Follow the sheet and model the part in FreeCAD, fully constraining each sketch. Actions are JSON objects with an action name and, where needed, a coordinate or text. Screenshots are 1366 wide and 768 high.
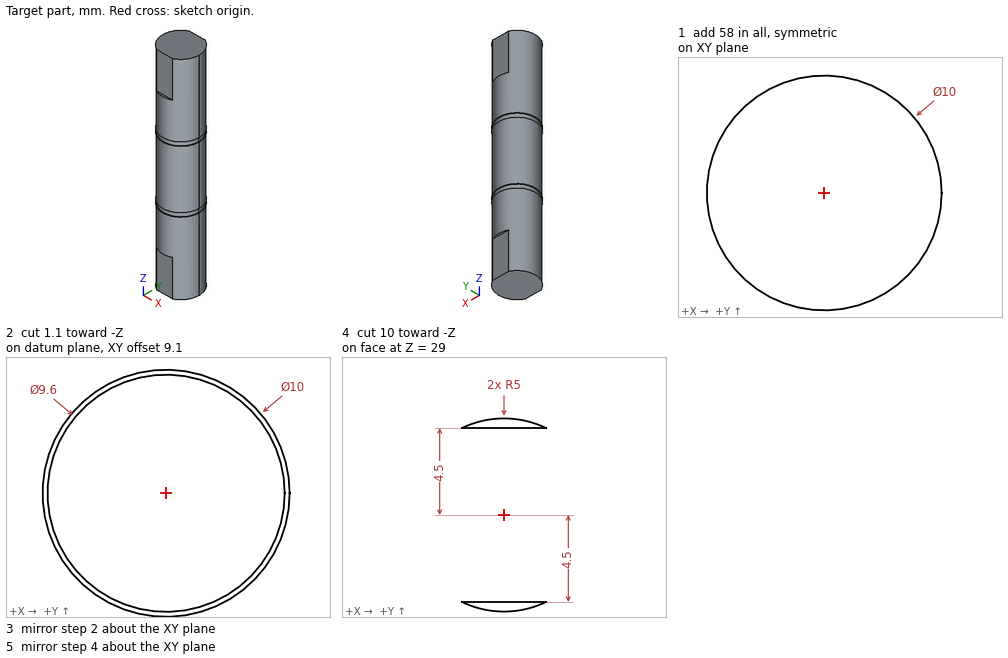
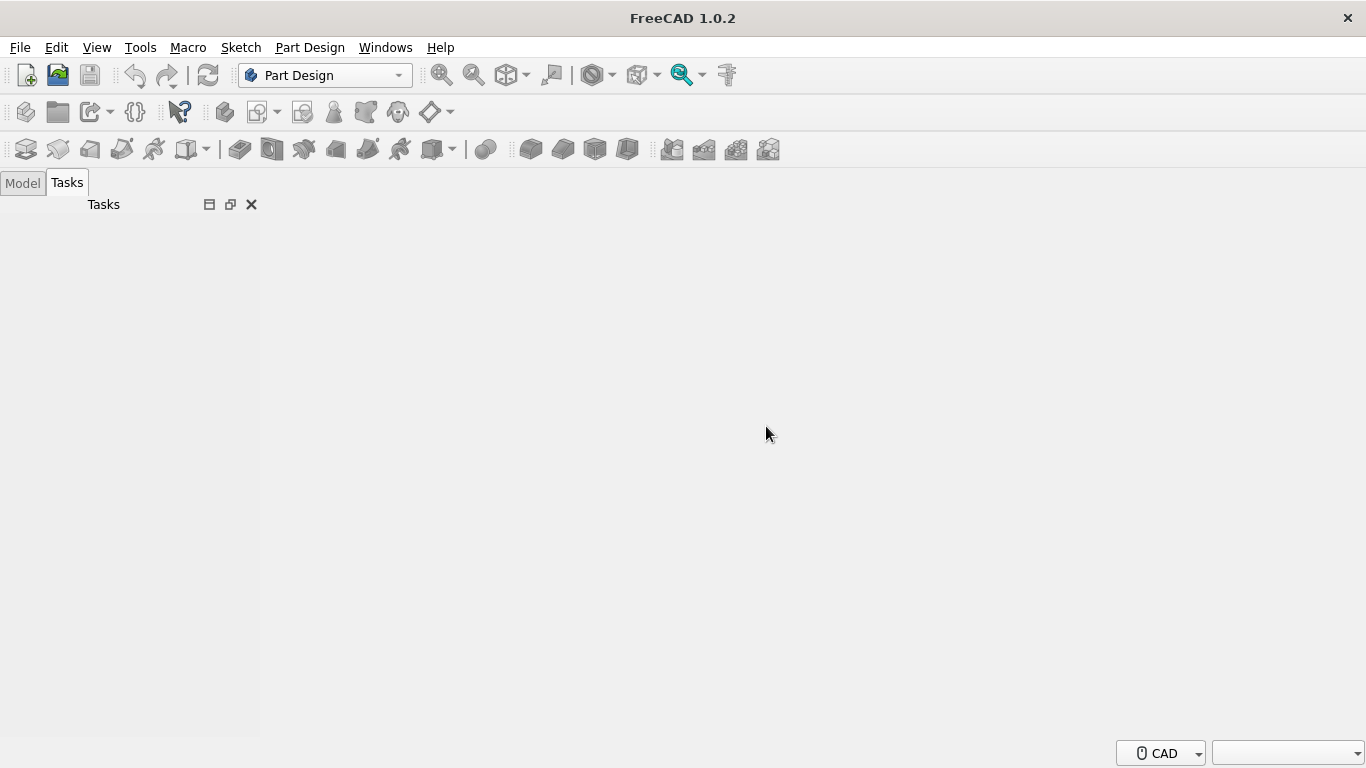
{"action": "key", "text": "ctrl+n"}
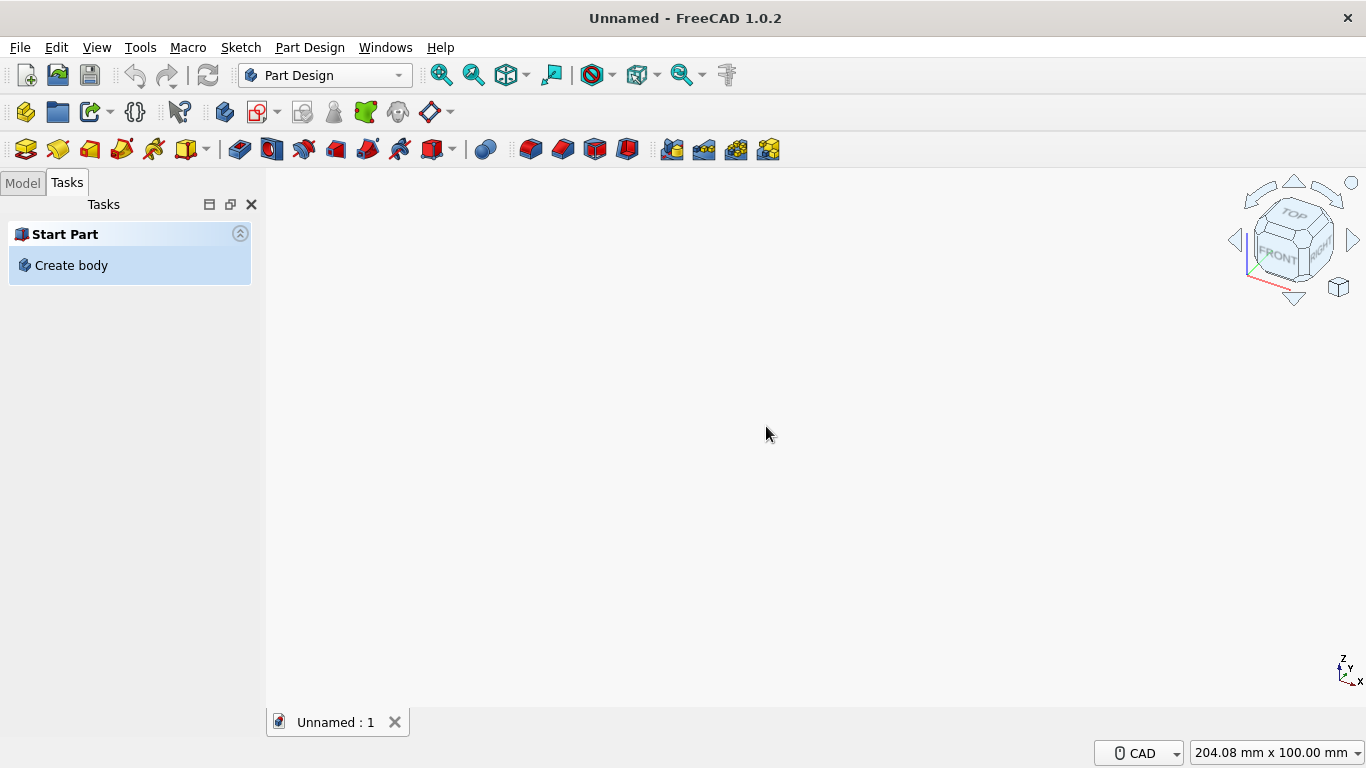
{"action": "left_click", "coordinate": [258, 112]}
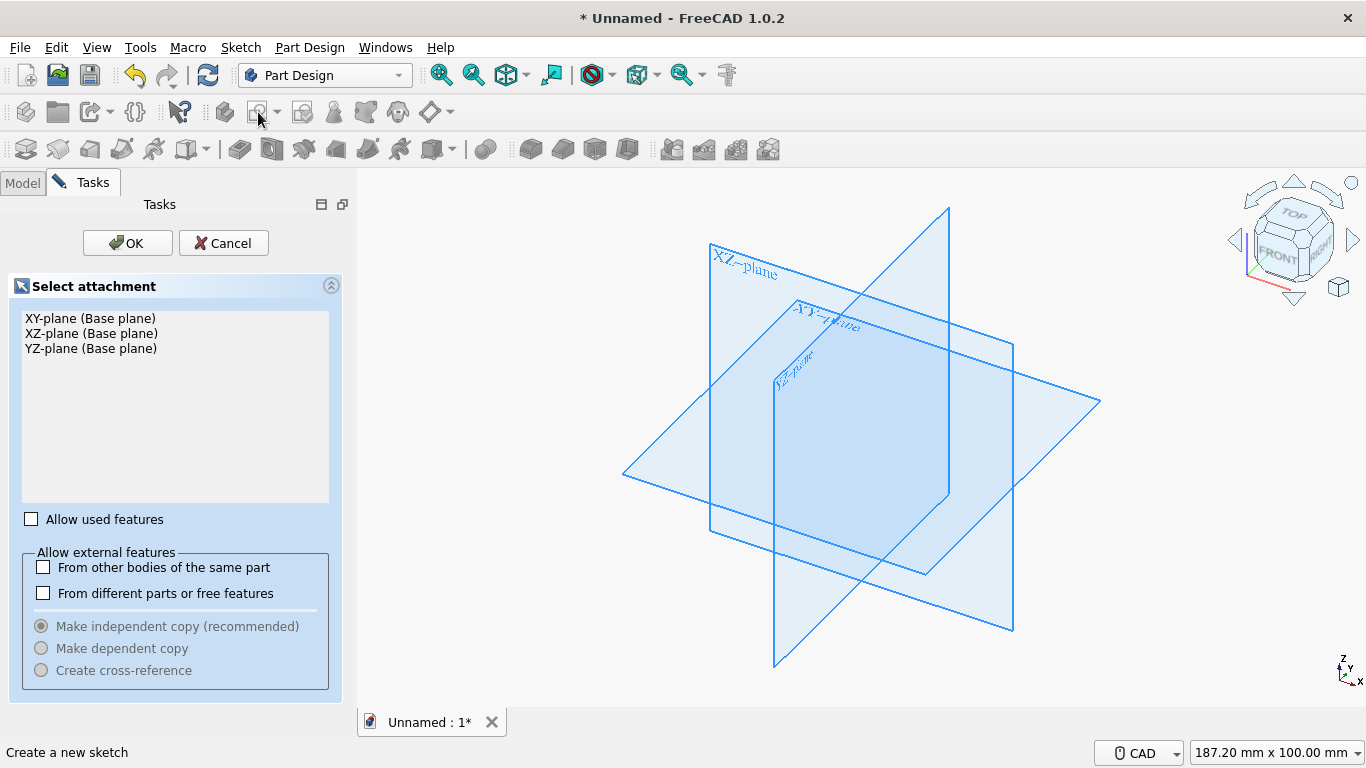
{"action": "left_click", "coordinate": [82, 318]}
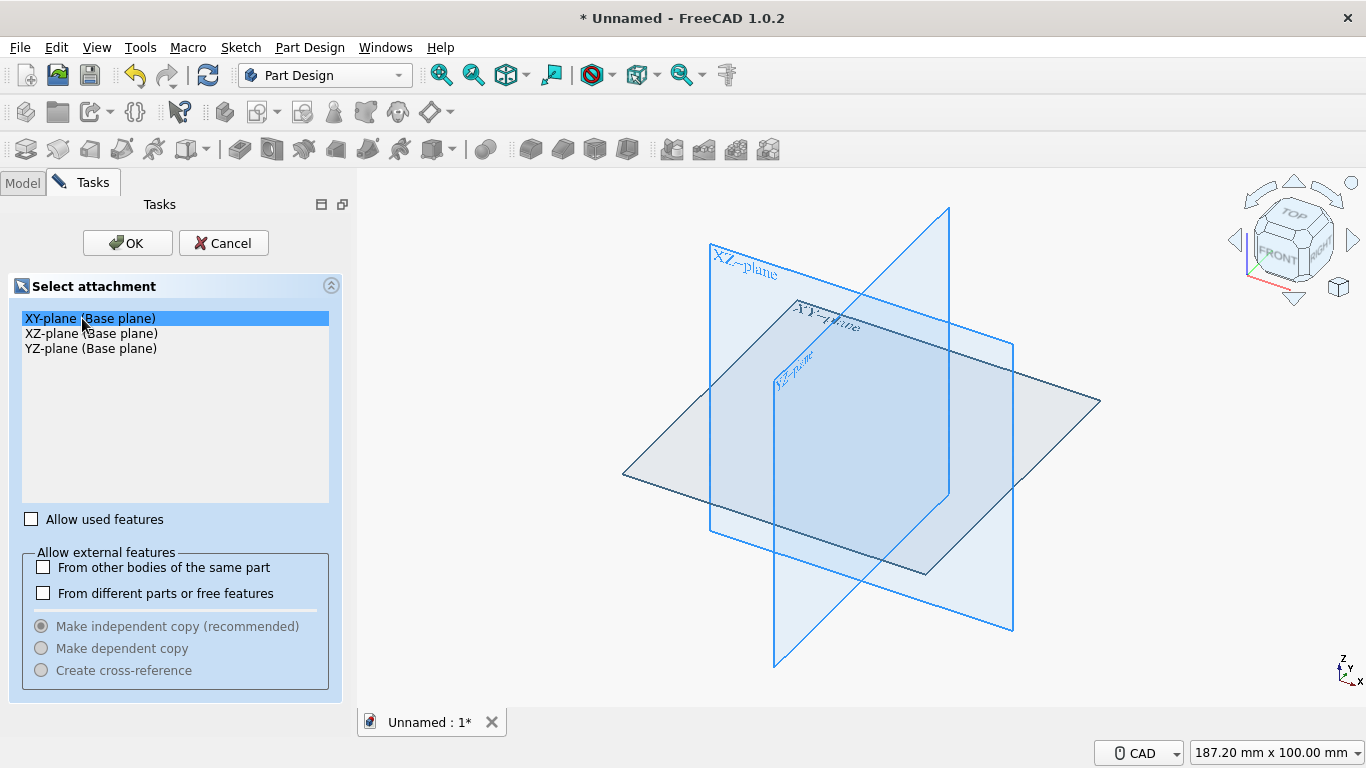
{"action": "left_click", "coordinate": [128, 243]}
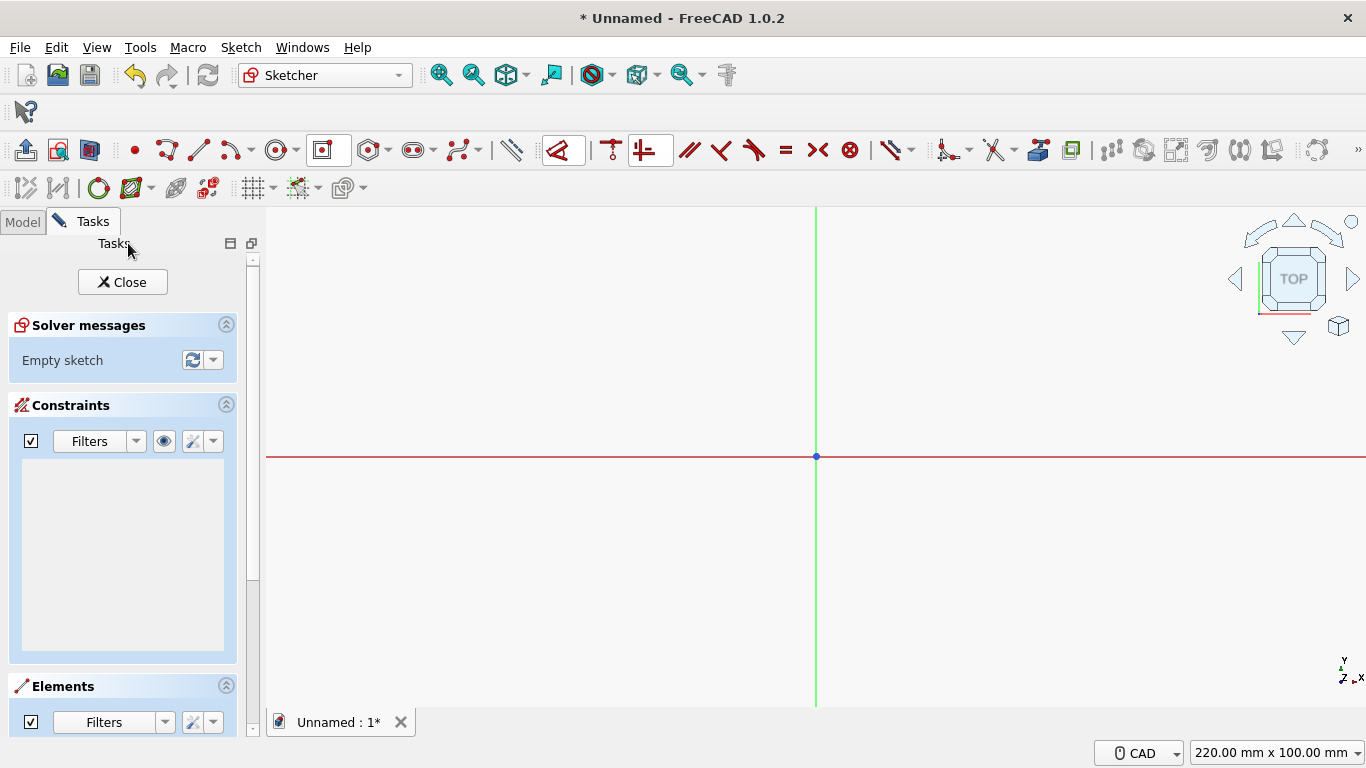
{"action": "scroll", "coordinate": [830, 457], "scroll_direction": "up", "scroll_amount": 9}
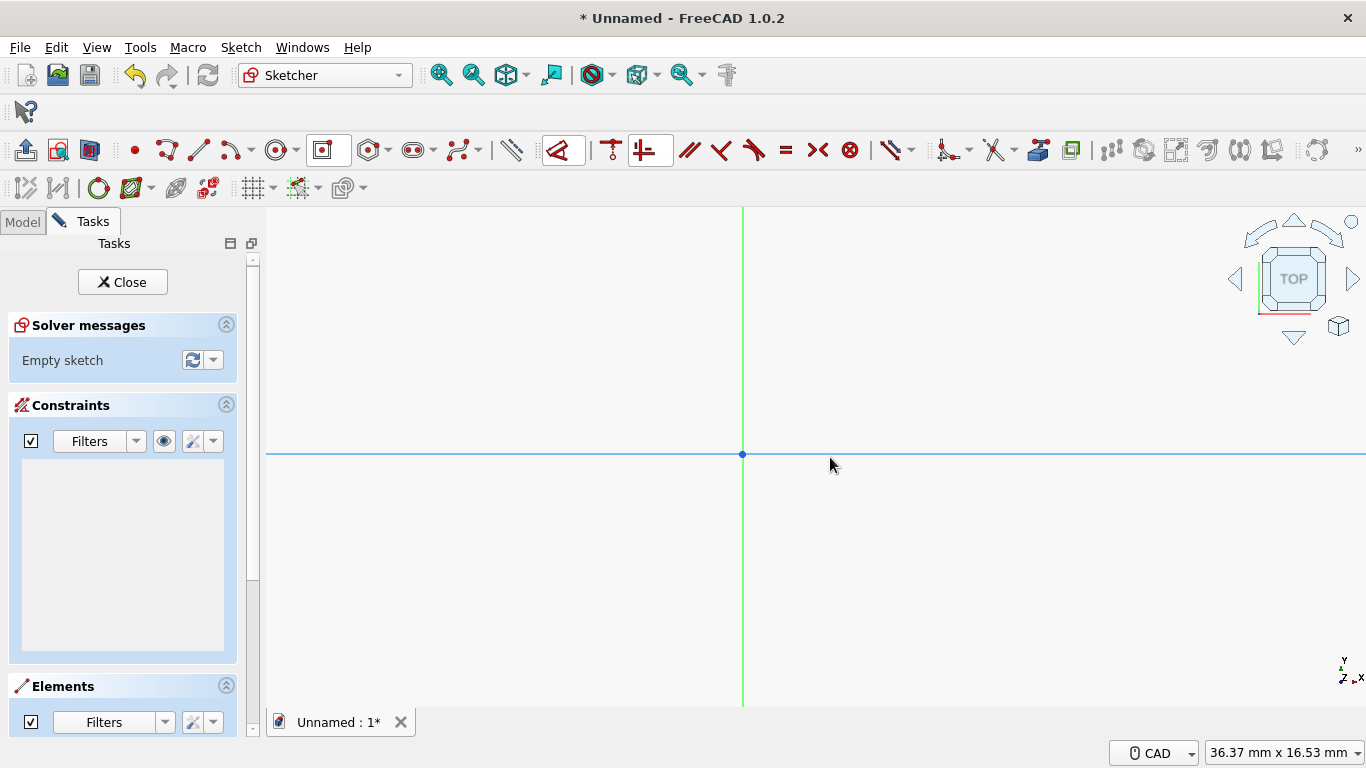
{"action": "left_click", "coordinate": [276, 150]}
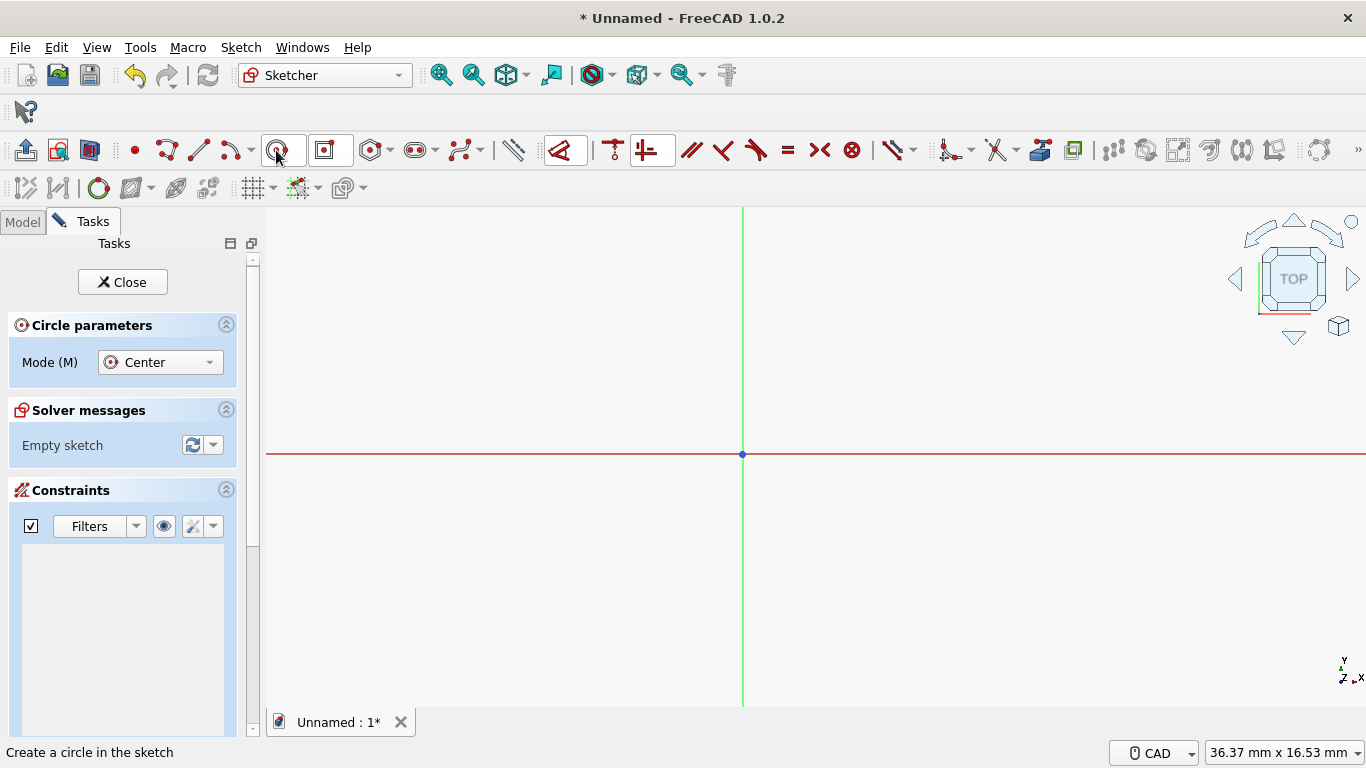
{"action": "left_click", "coordinate": [743, 454]}
{"action": "left_click", "coordinate": [850, 348]}
{"action": "key", "text": "Escape"}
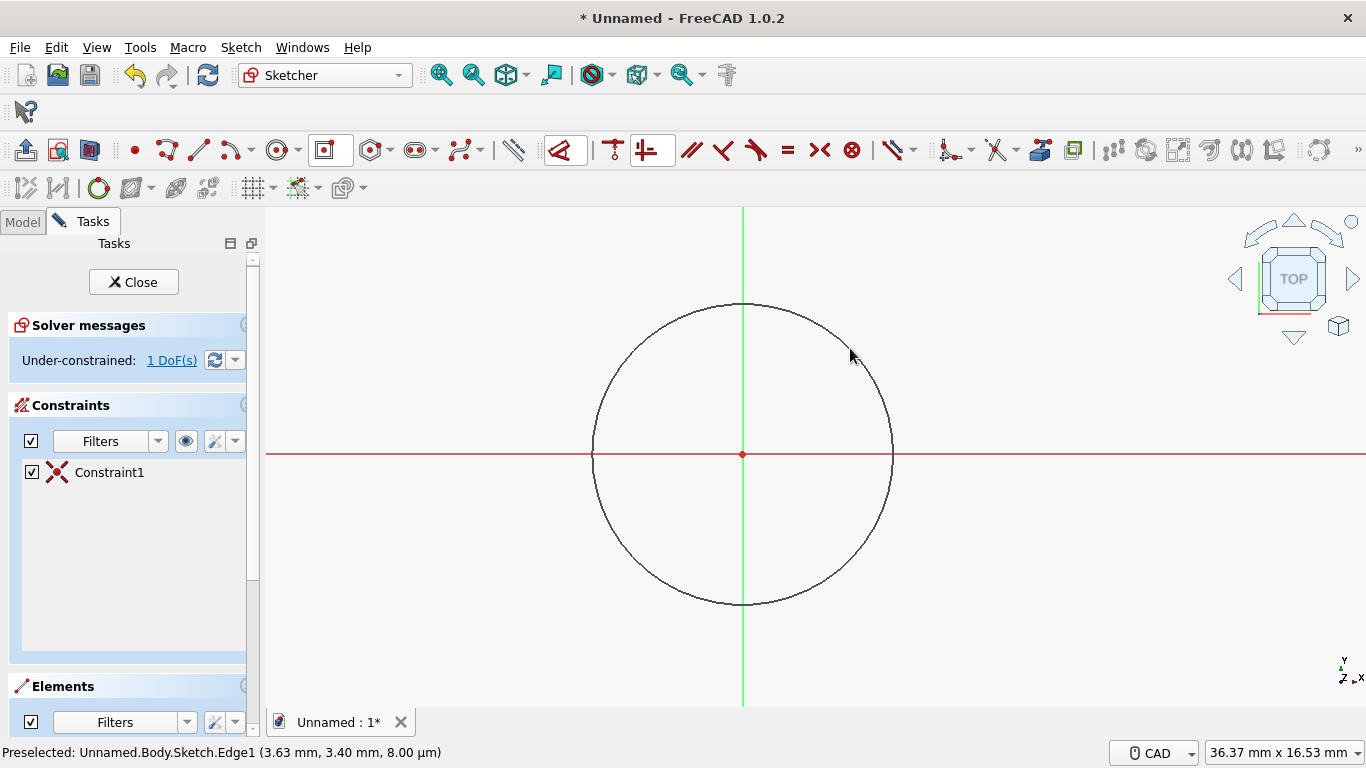
{"action": "left_click", "coordinate": [560, 150]}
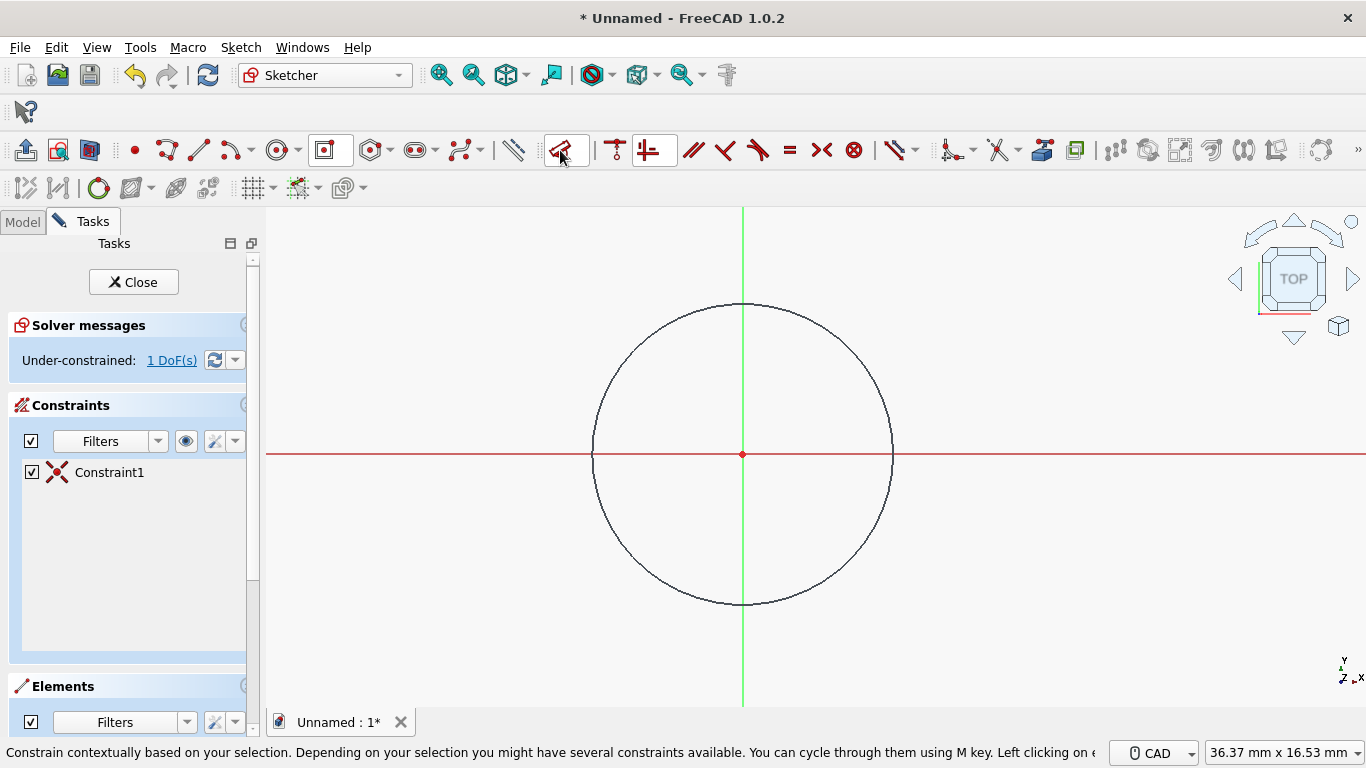
{"action": "left_click", "coordinate": [849, 348]}
{"action": "left_click", "coordinate": [872, 325]}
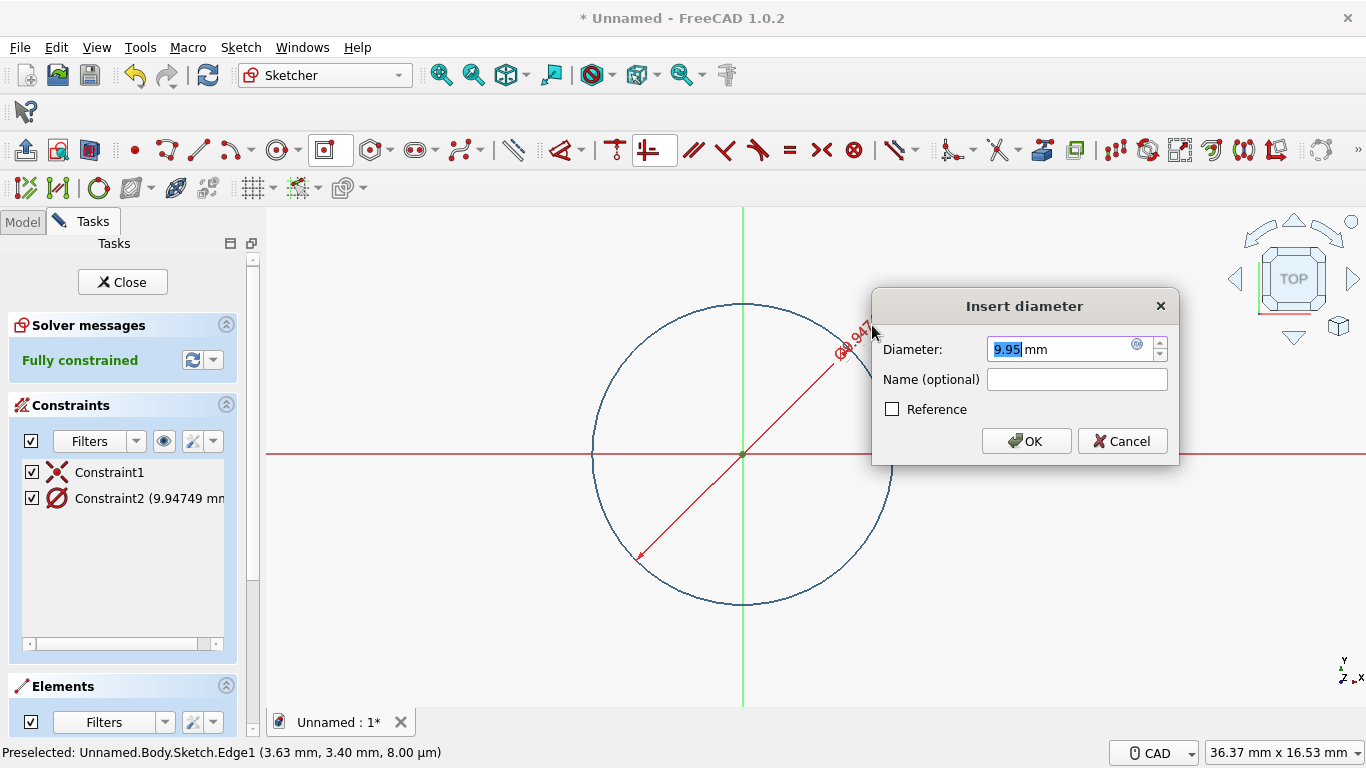
{"action": "type", "text": "10"}
{"action": "key", "text": "Return"}
{"action": "key", "text": "Escape"}